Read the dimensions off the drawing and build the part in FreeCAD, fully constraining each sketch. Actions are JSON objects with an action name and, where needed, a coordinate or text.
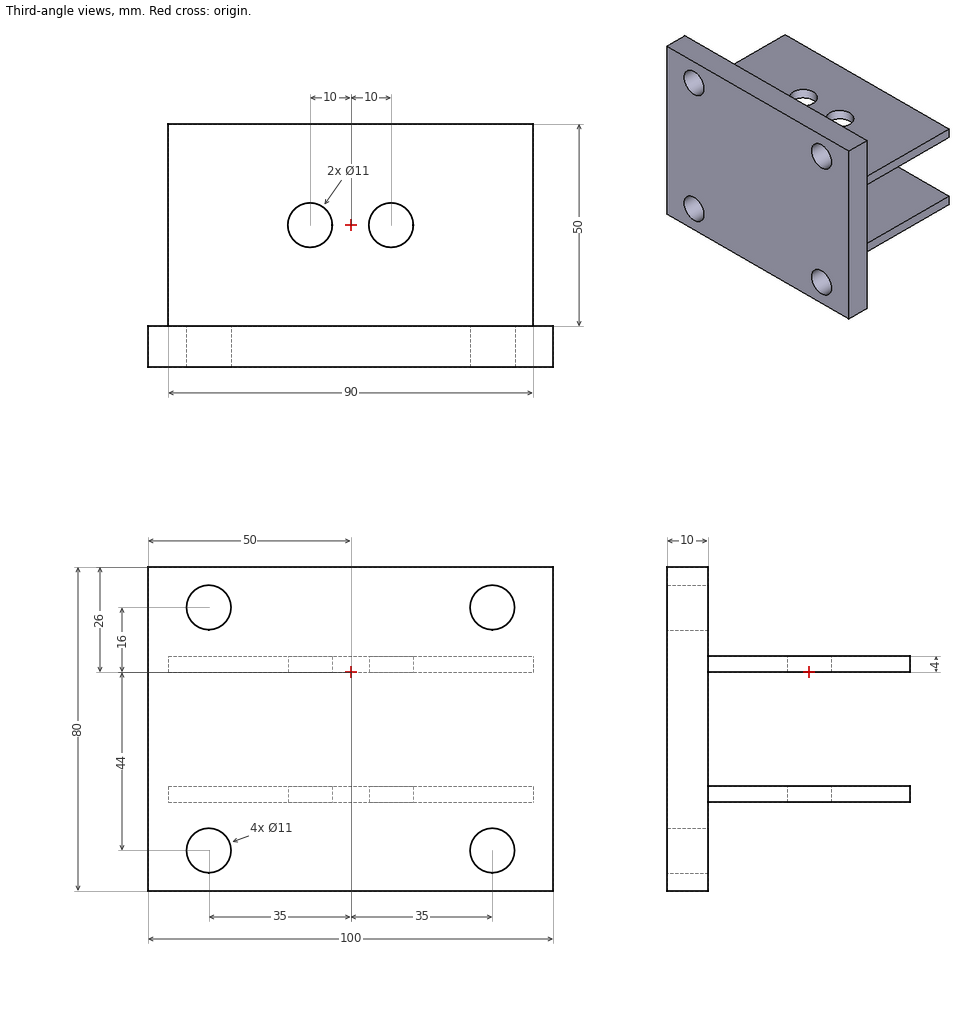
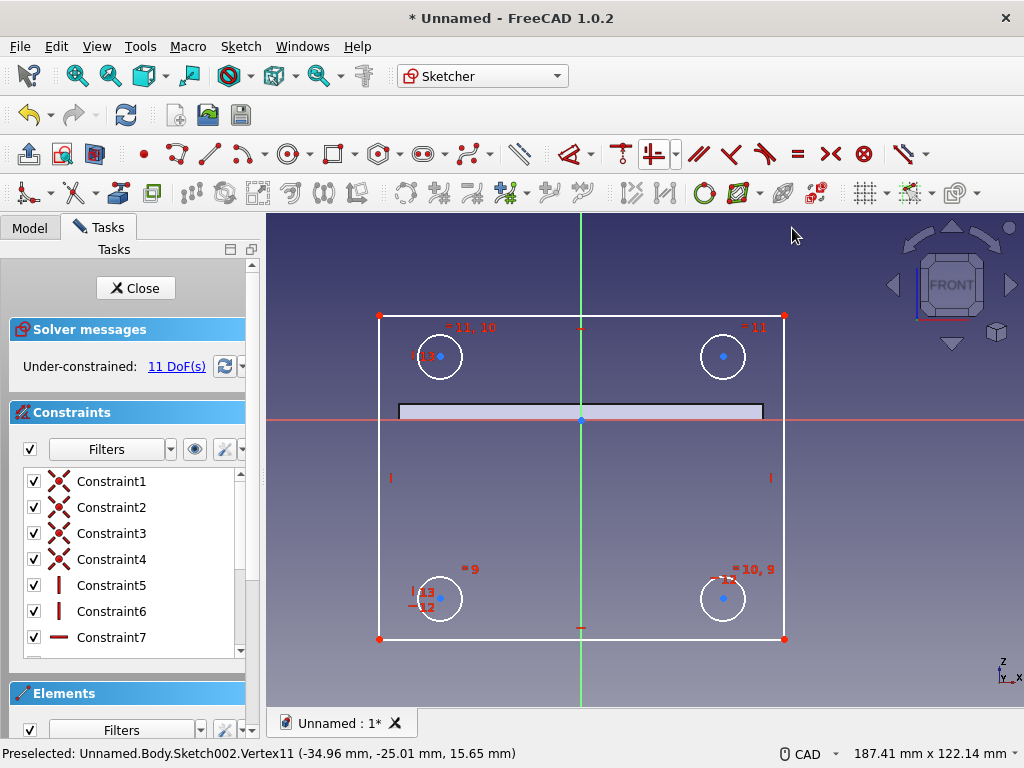
{"action": "left_click", "coordinate": [723, 599]}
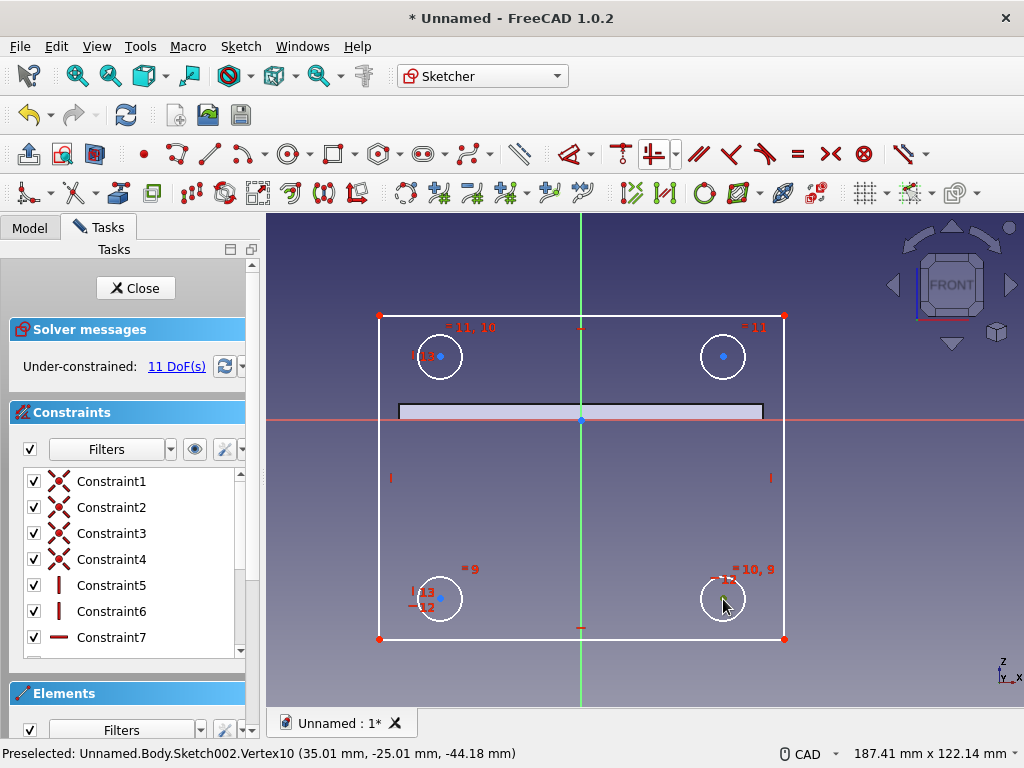
{"action": "left_click", "coordinate": [723, 357]}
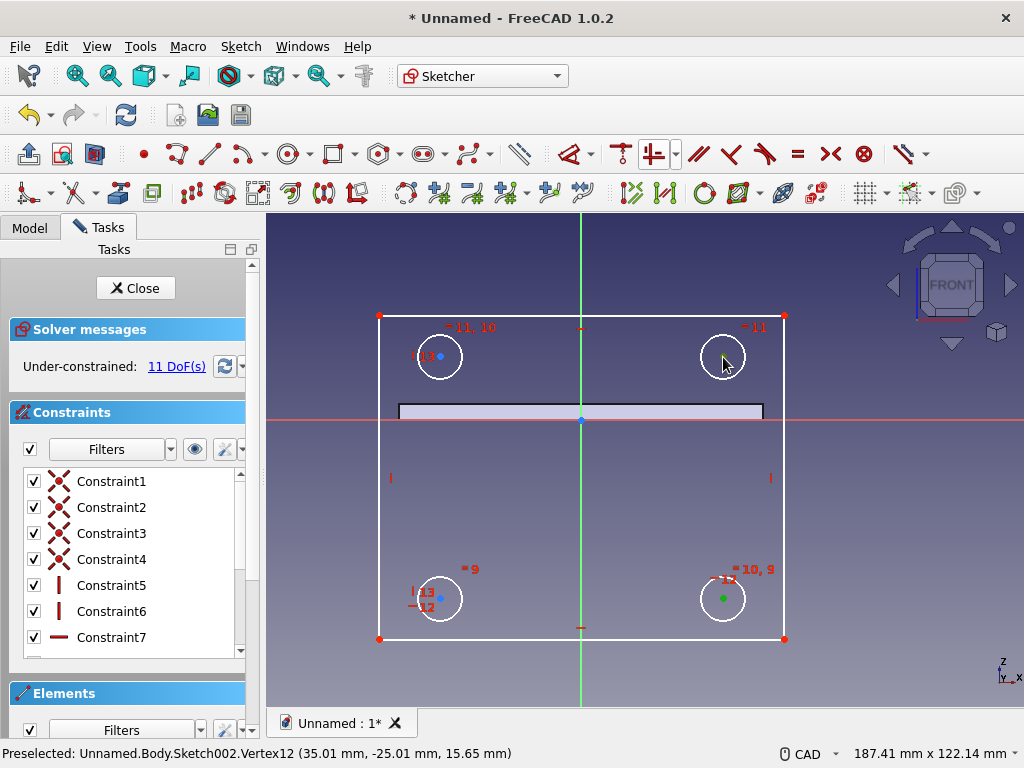
{"action": "key", "text": "v"}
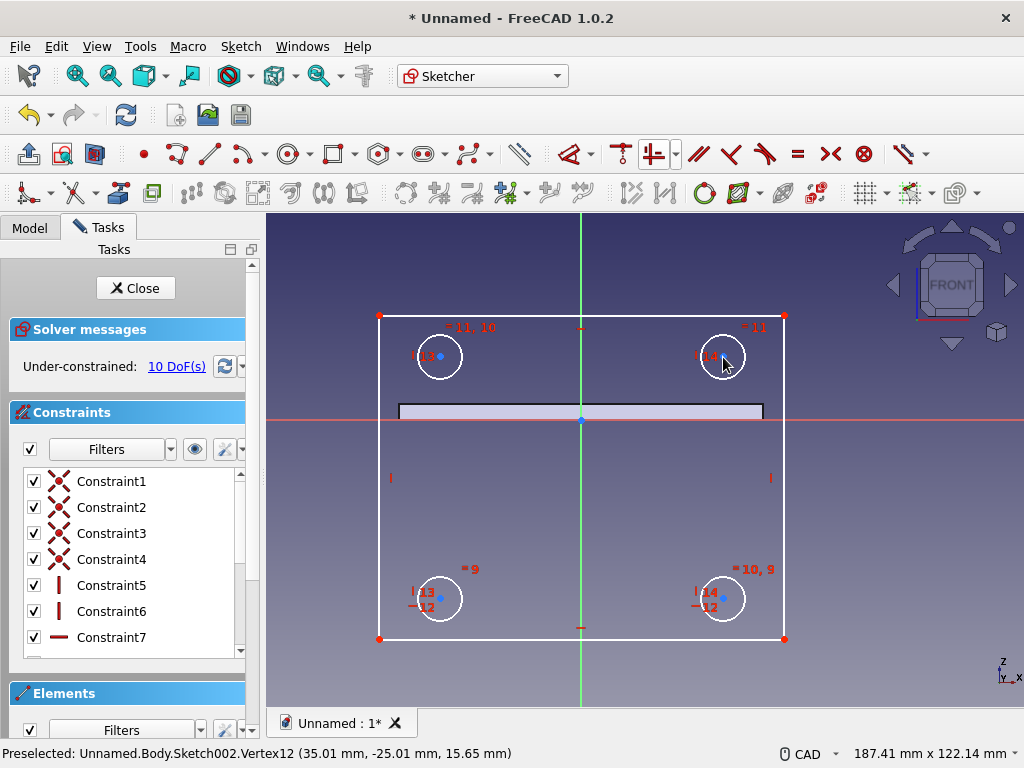
{"action": "left_click", "coordinate": [440, 357]}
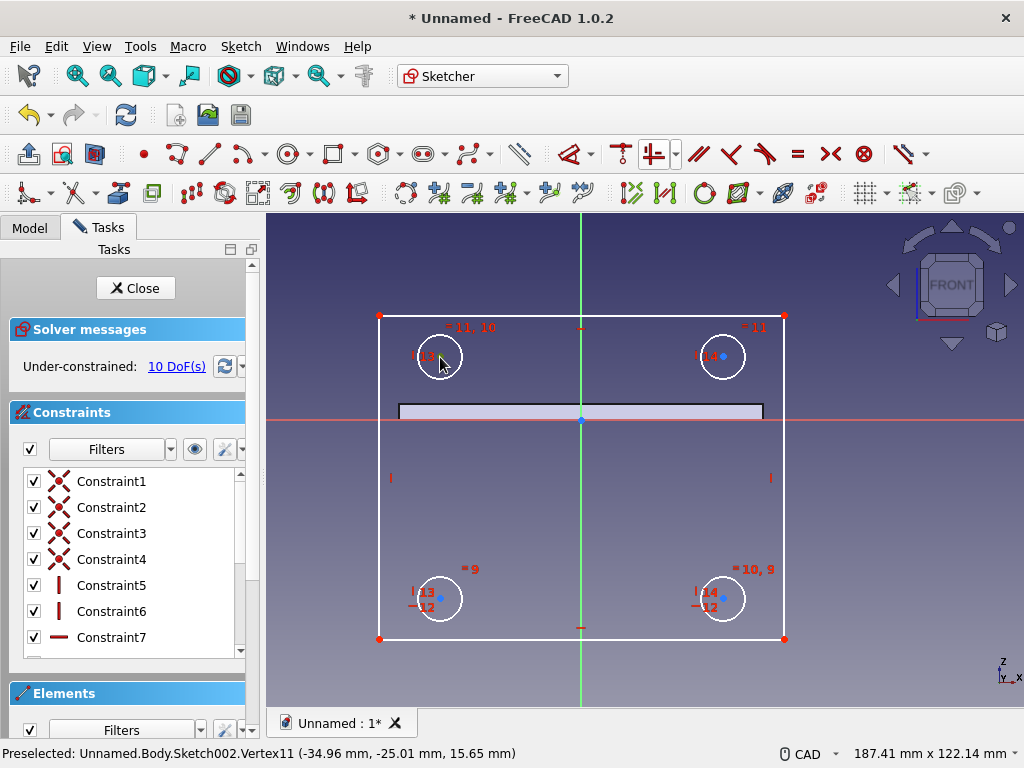
{"action": "left_click", "coordinate": [723, 357]}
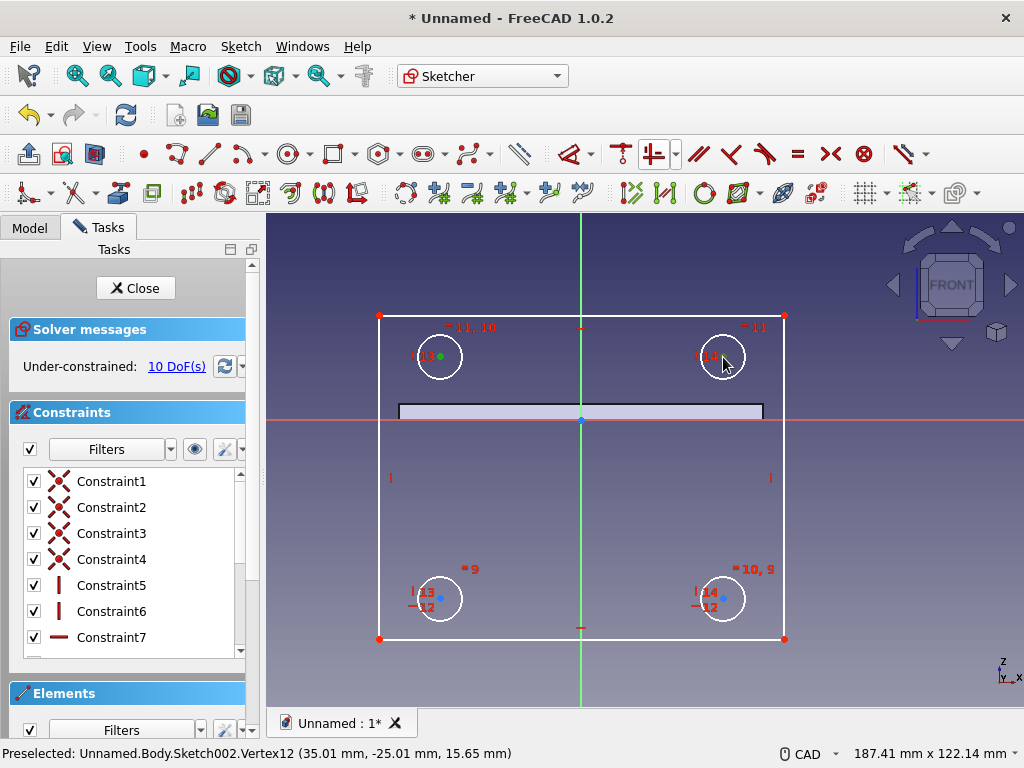
{"action": "left_click", "coordinate": [676, 154]}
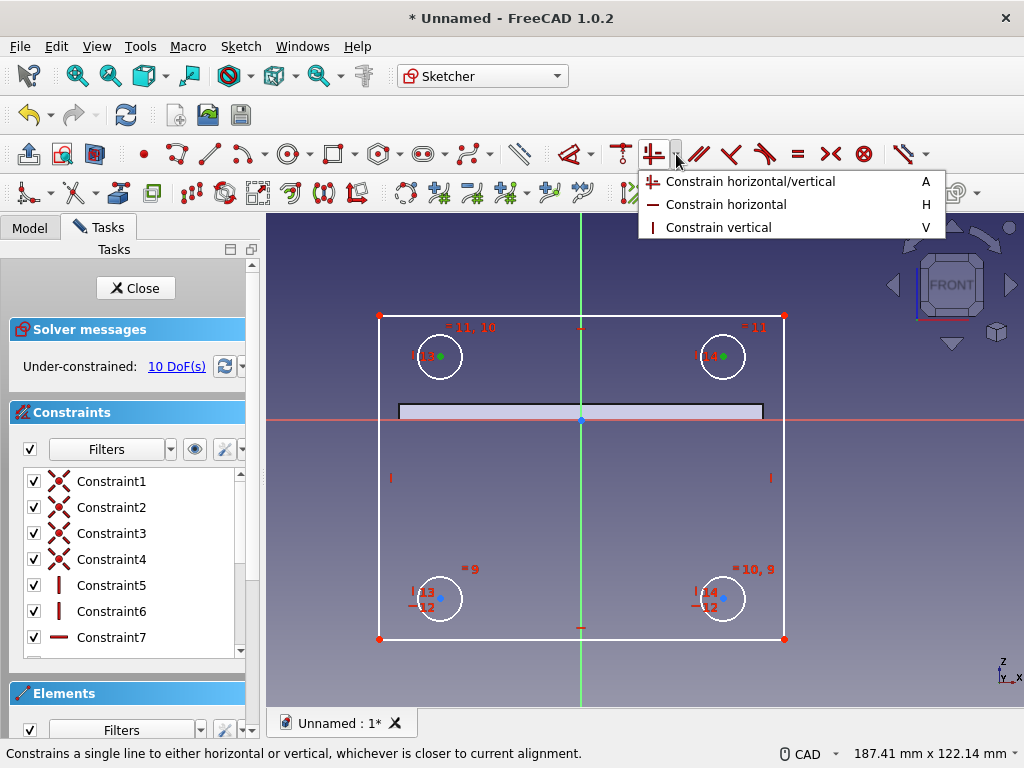
{"action": "left_click", "coordinate": [792, 204]}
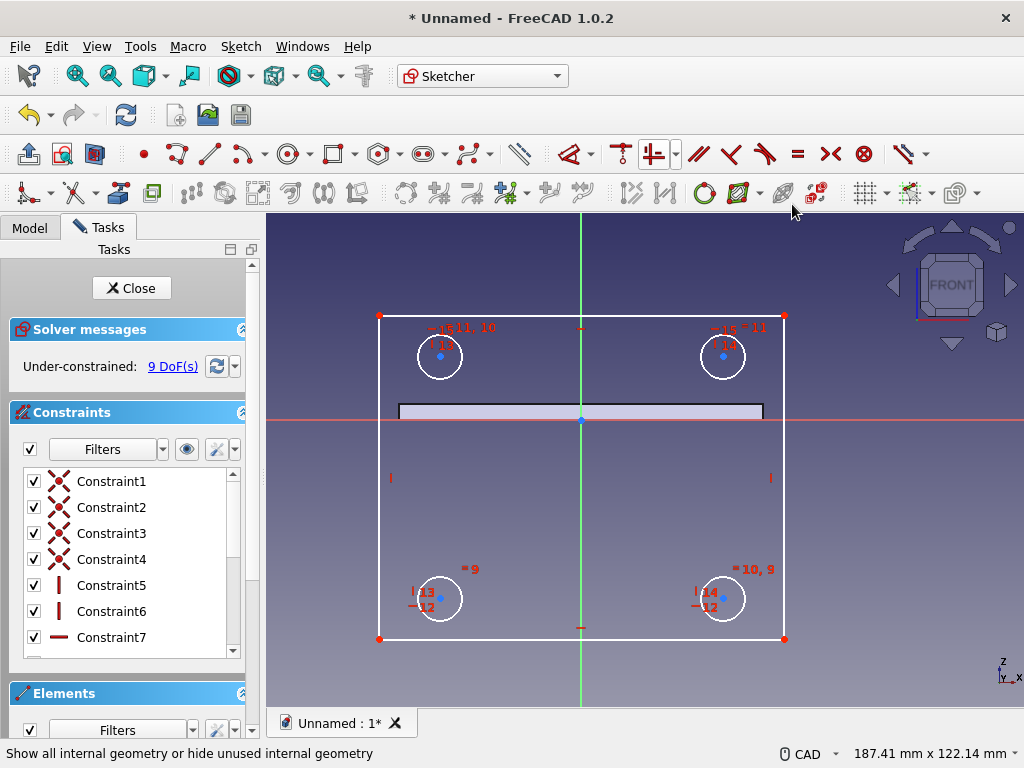
{"action": "key", "text": "d"}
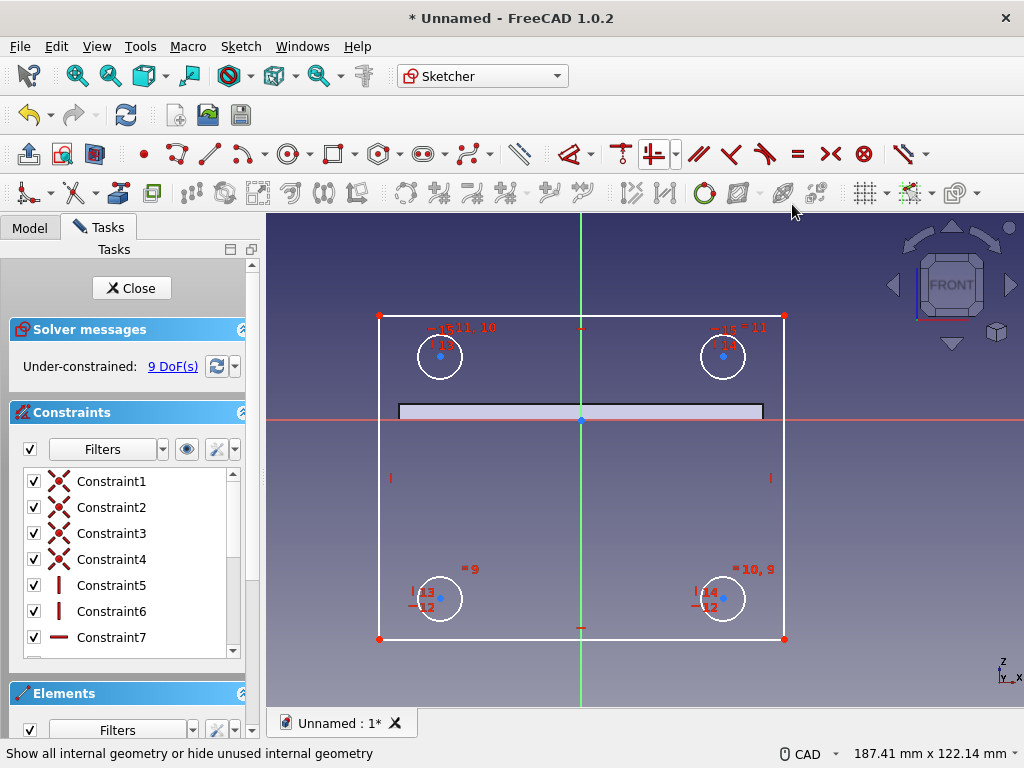
{"action": "left_click", "coordinate": [455, 583]}
{"action": "left_click", "coordinate": [477, 560]}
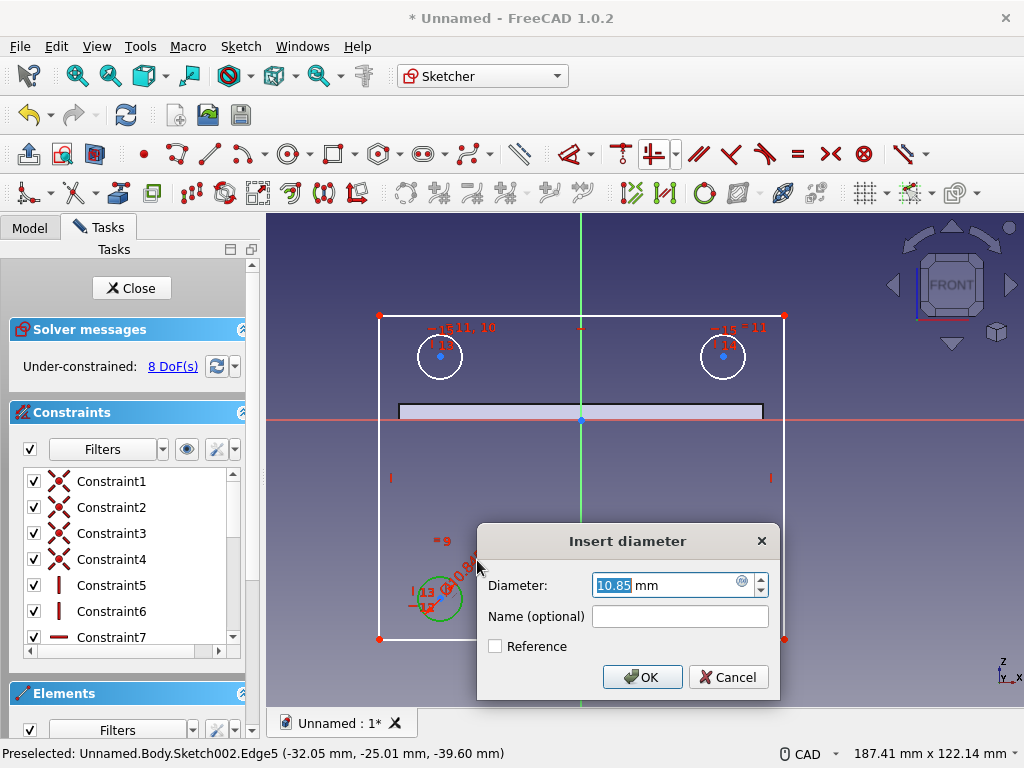
{"action": "type", "text": "11"}
{"action": "key", "text": "Return"}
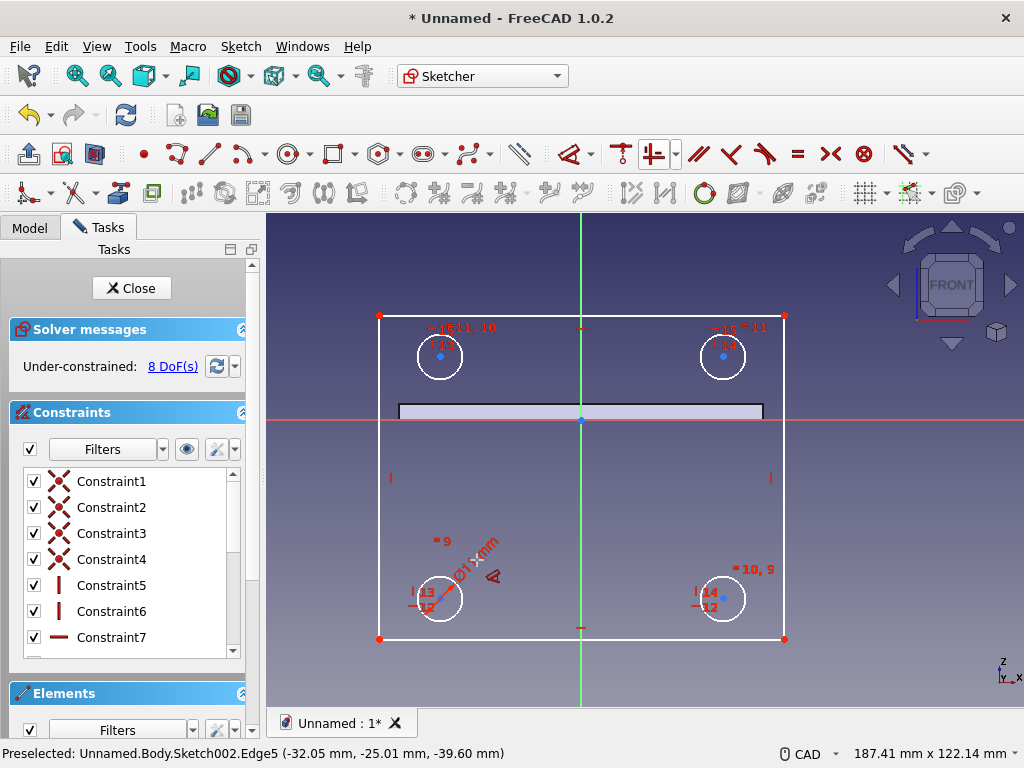
{"action": "left_click", "coordinate": [379, 543]}
{"action": "left_click", "coordinate": [345, 478]}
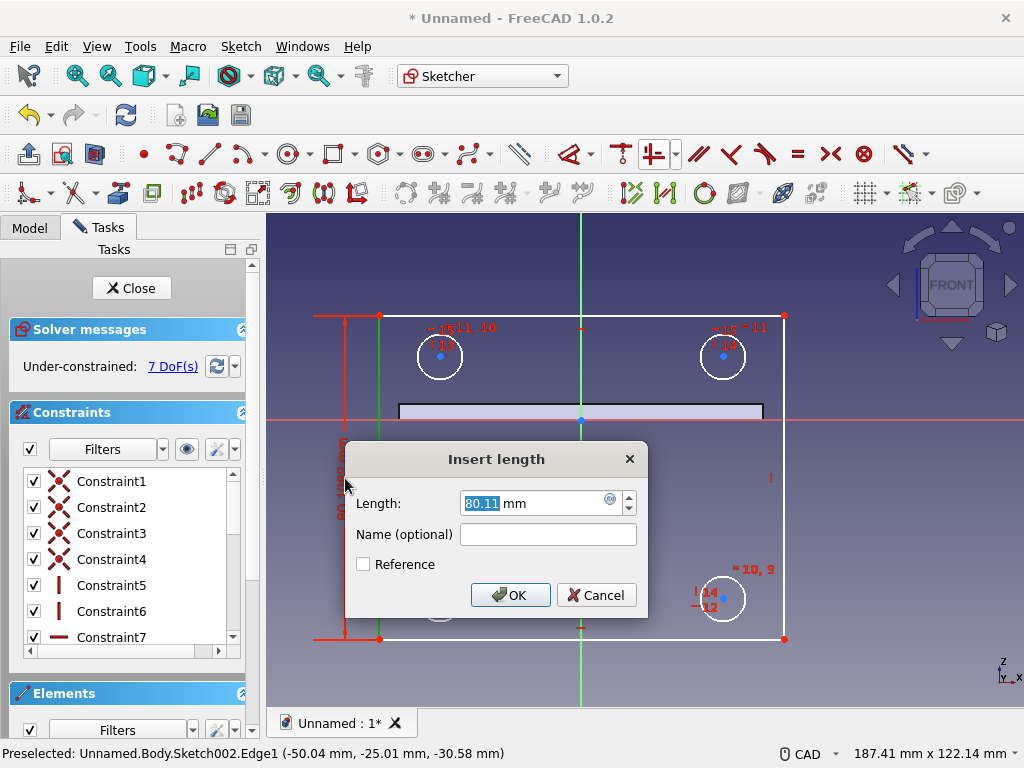
{"action": "type", "text": "80"}
{"action": "key", "text": "Return"}